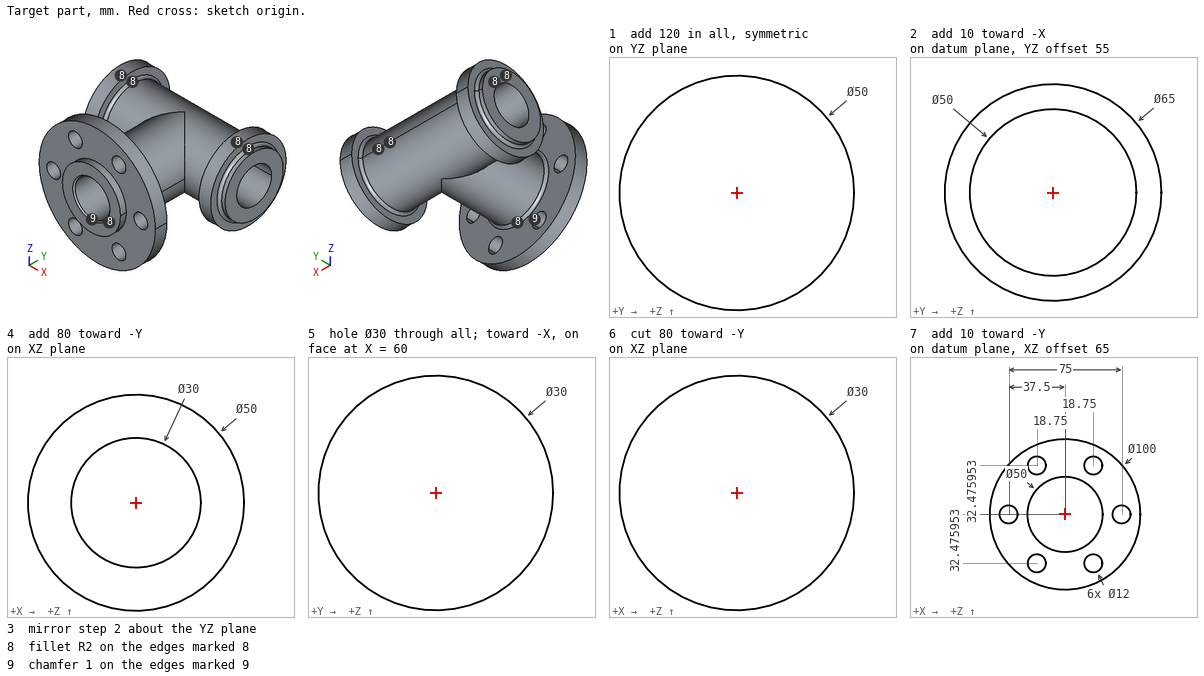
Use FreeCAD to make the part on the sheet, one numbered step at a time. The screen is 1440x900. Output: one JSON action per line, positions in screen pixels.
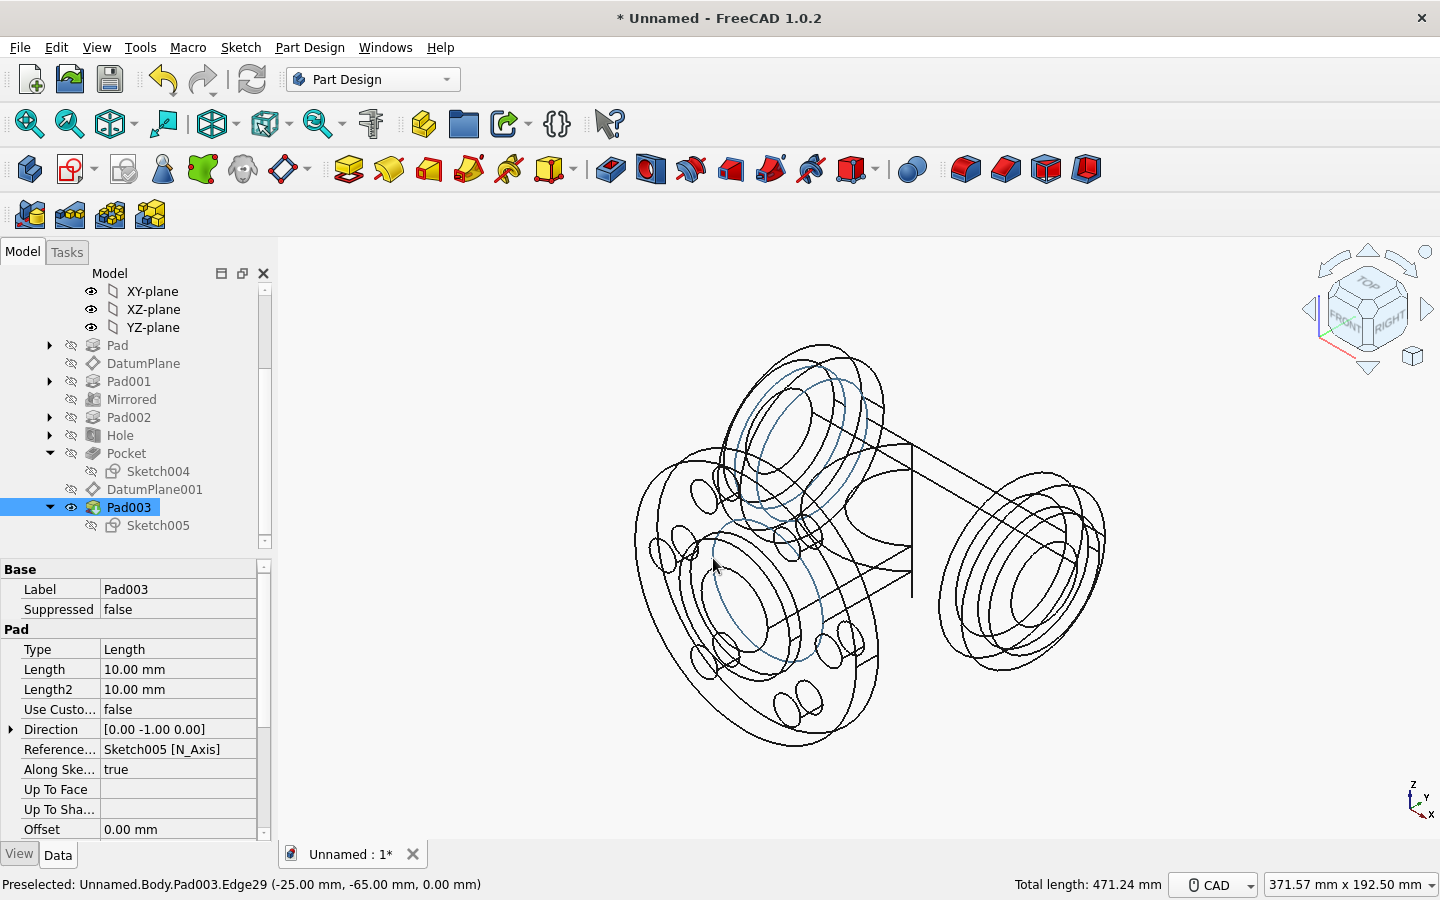
{"action": "left_click", "coordinate": [956, 596], "text": "ctrl"}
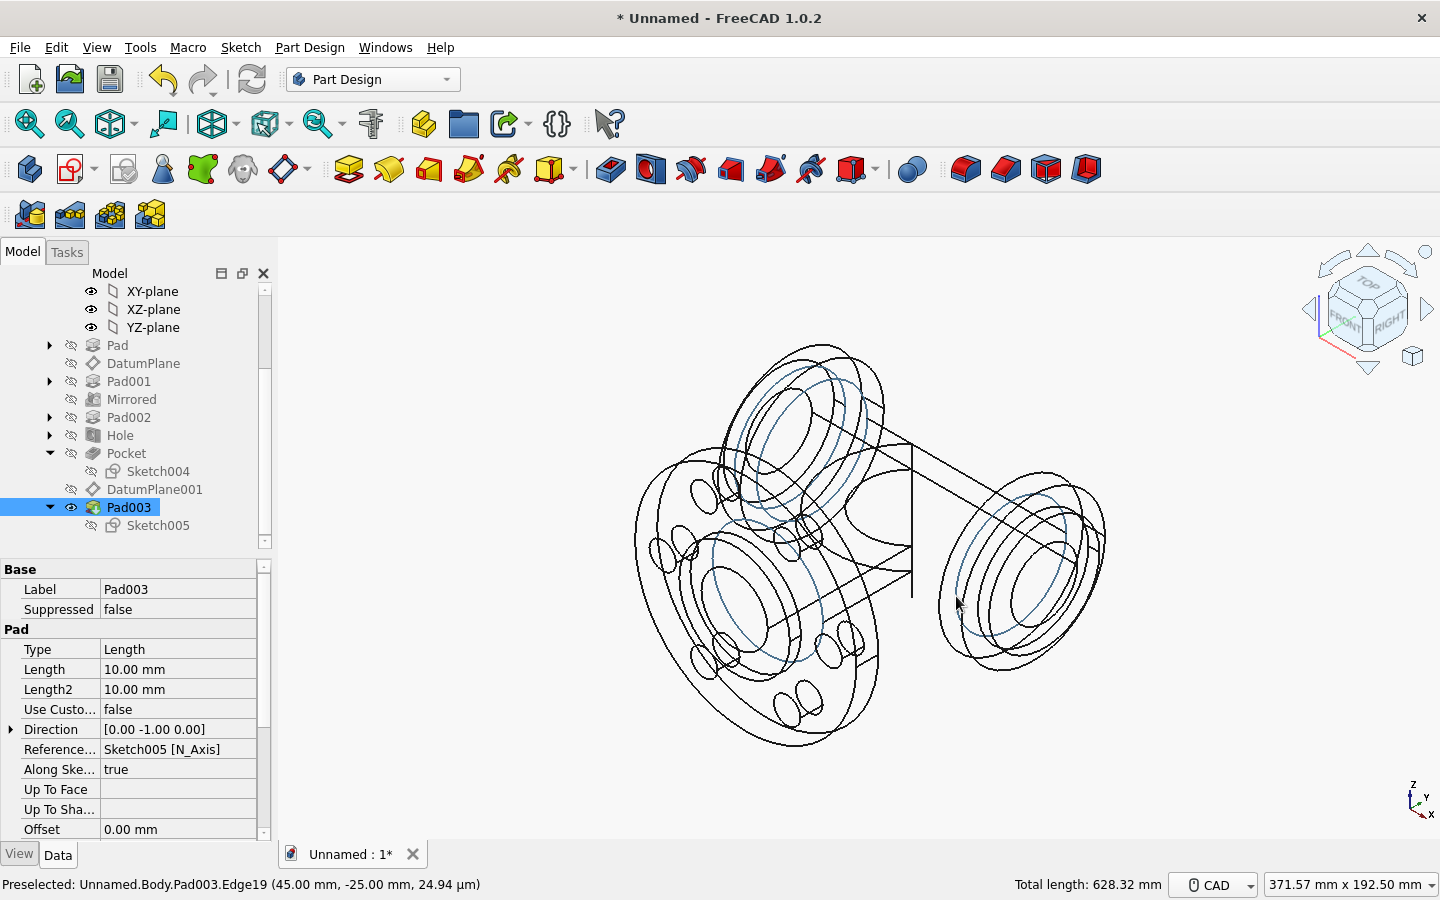
{"action": "left_click", "coordinate": [978, 609], "text": "ctrl"}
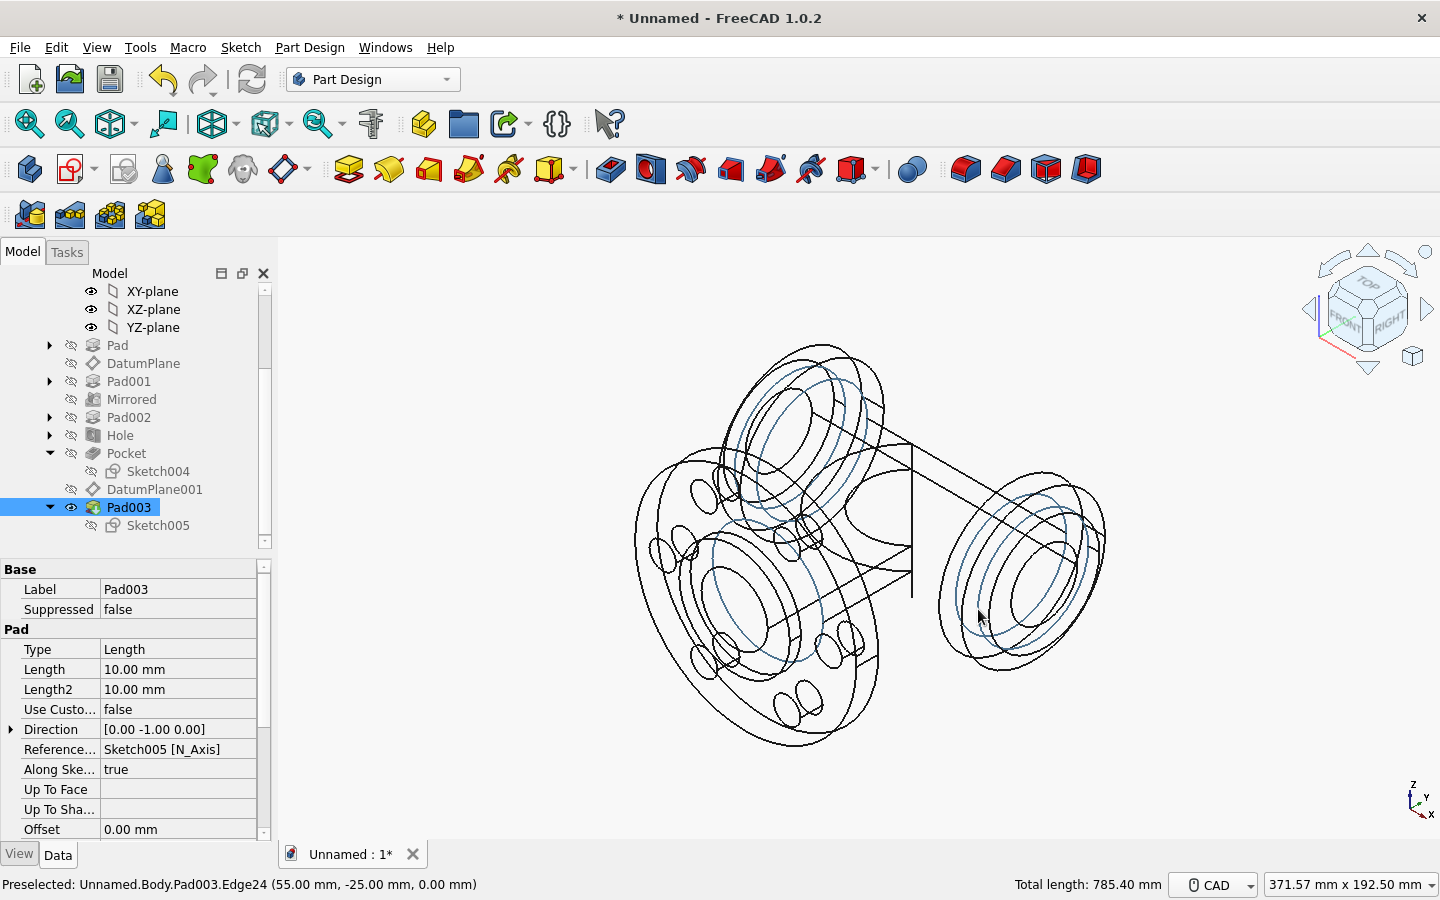
{"action": "key", "text": "v 1"}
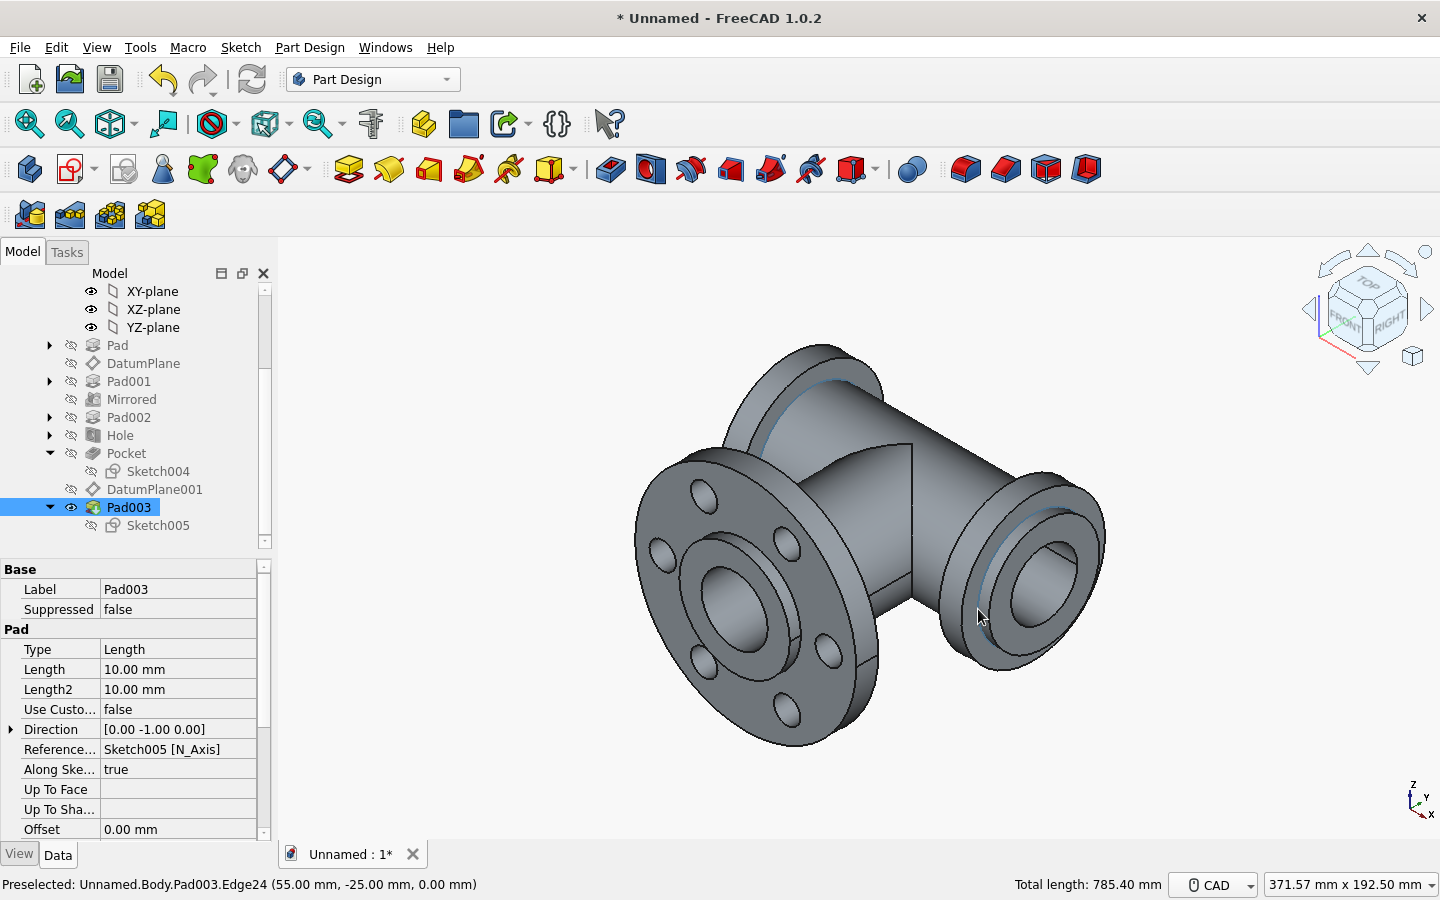
{"action": "left_click", "coordinate": [966, 170]}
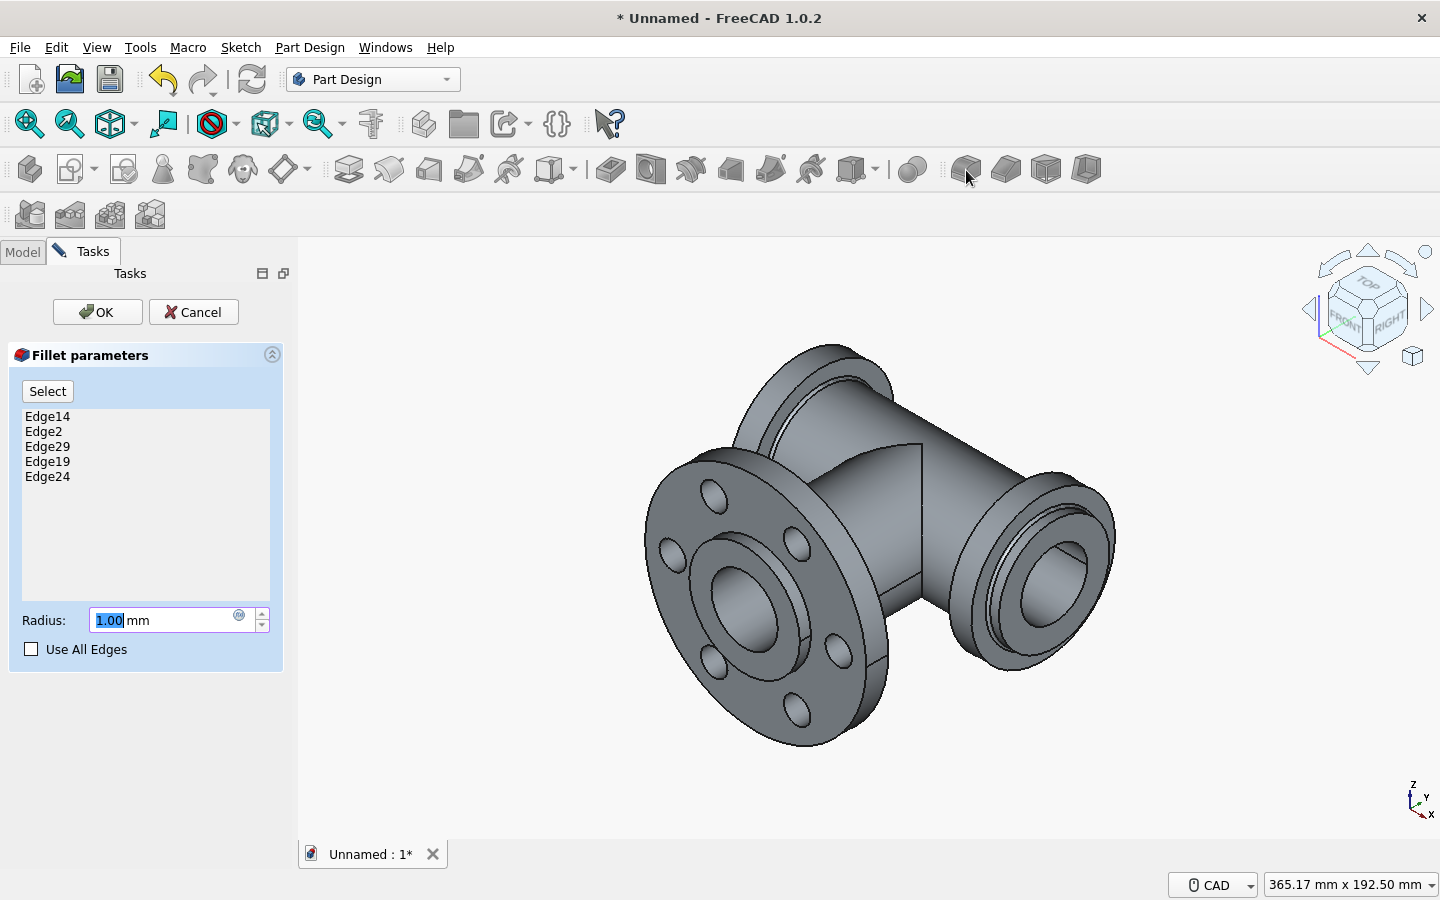
{"action": "type", "text": "2"}
{"action": "key", "text": "Tab"}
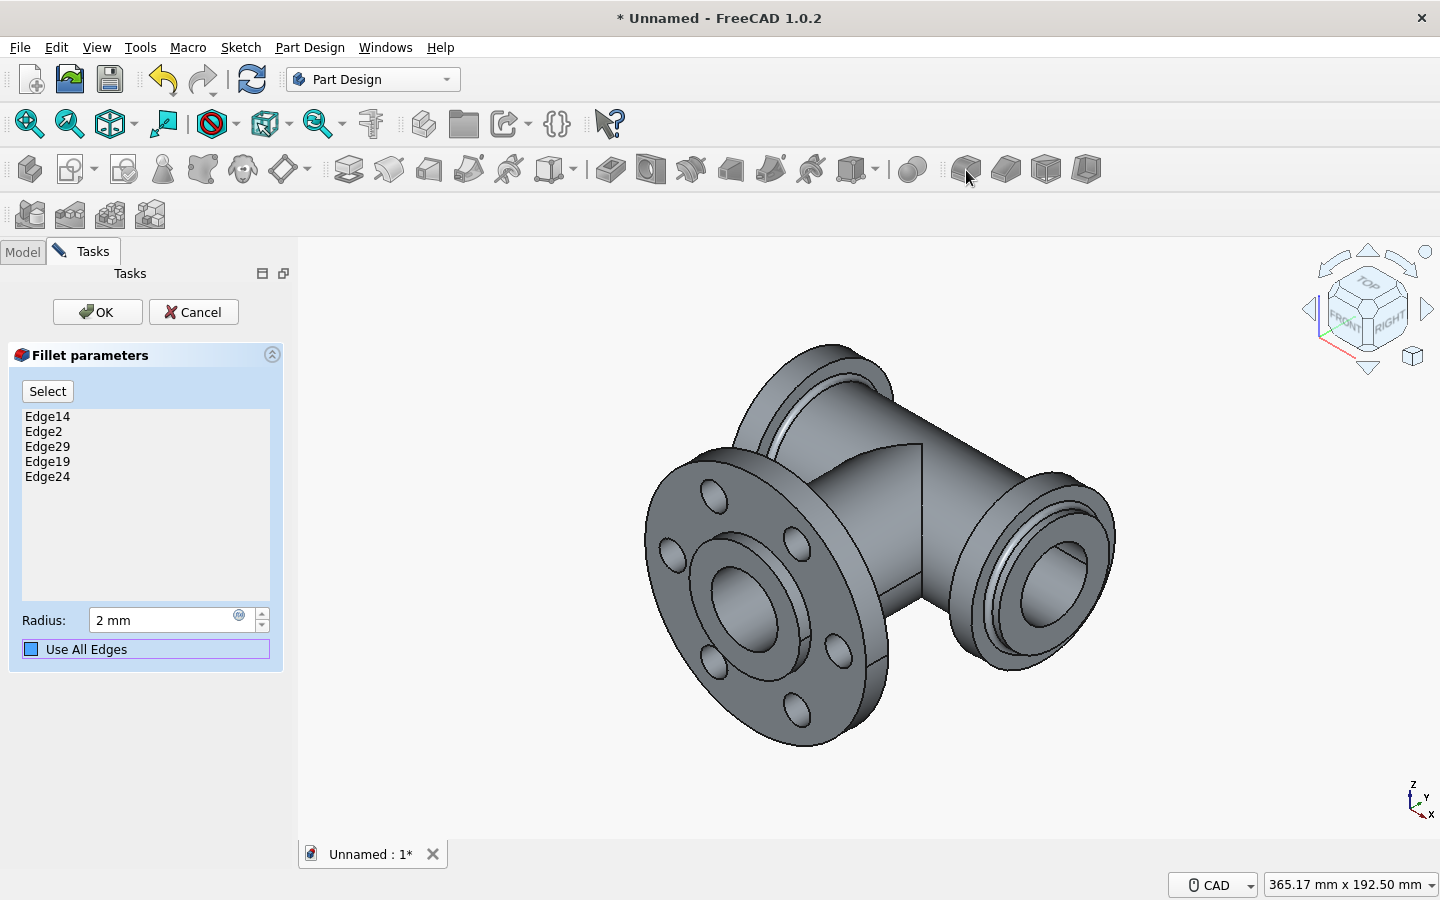
{"action": "left_click", "coordinate": [98, 312]}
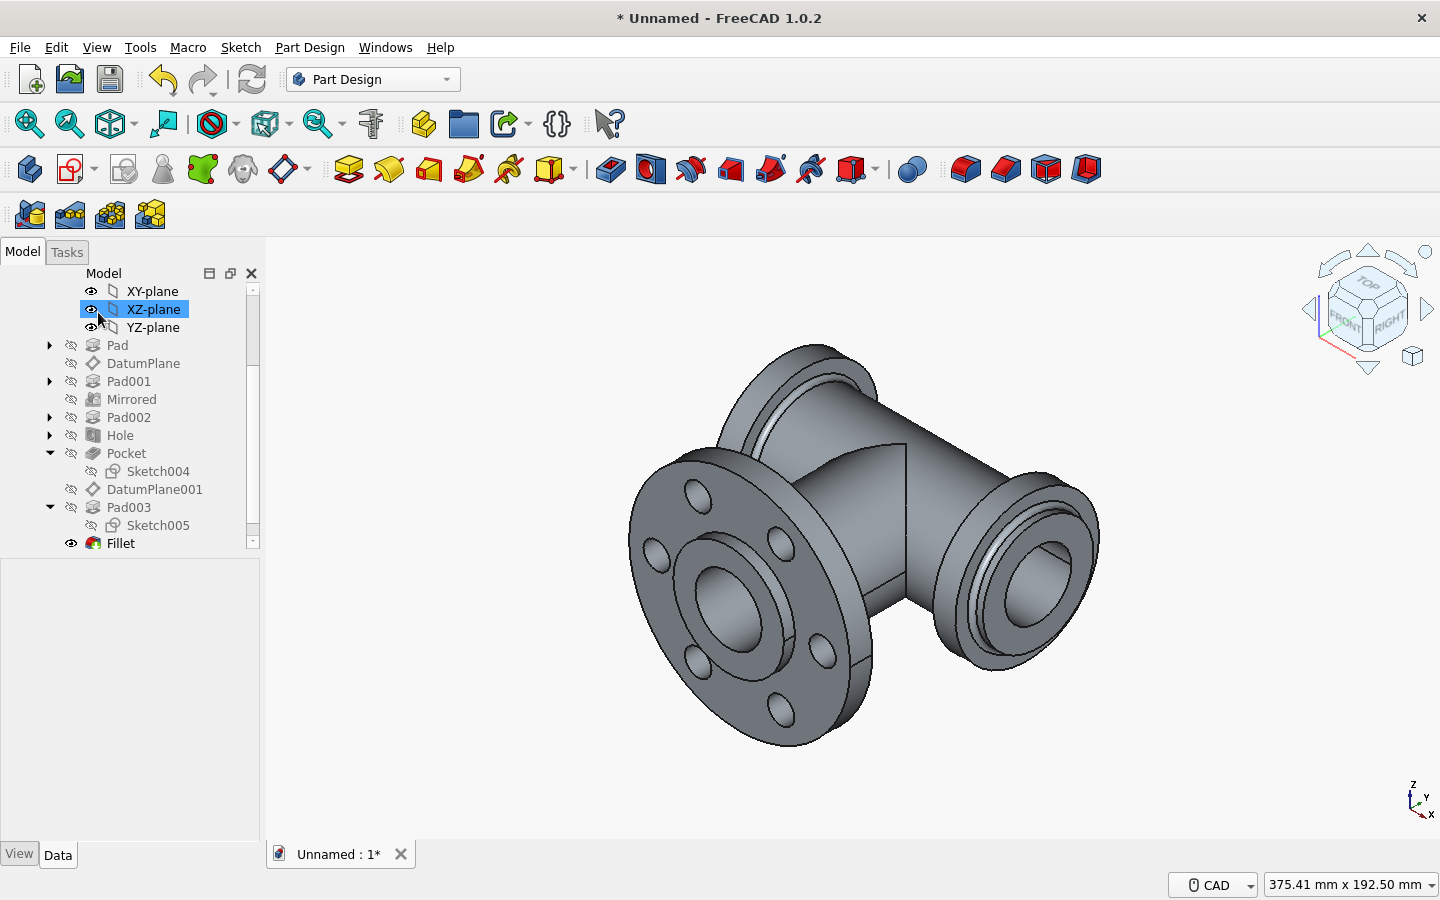
{"action": "left_click", "coordinate": [695, 590]}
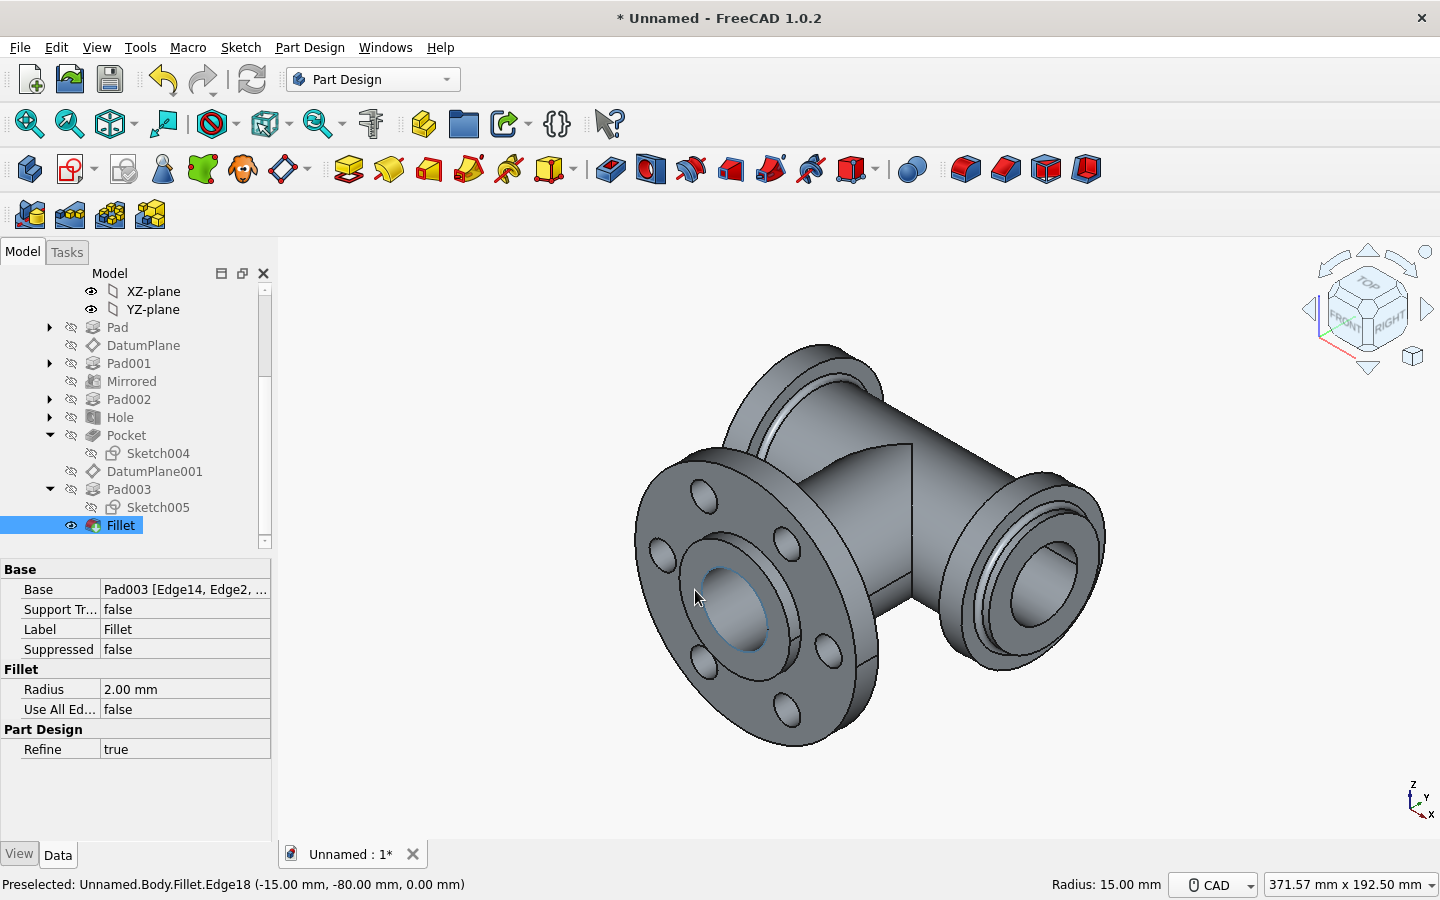
{"action": "left_click", "coordinate": [1006, 170]}